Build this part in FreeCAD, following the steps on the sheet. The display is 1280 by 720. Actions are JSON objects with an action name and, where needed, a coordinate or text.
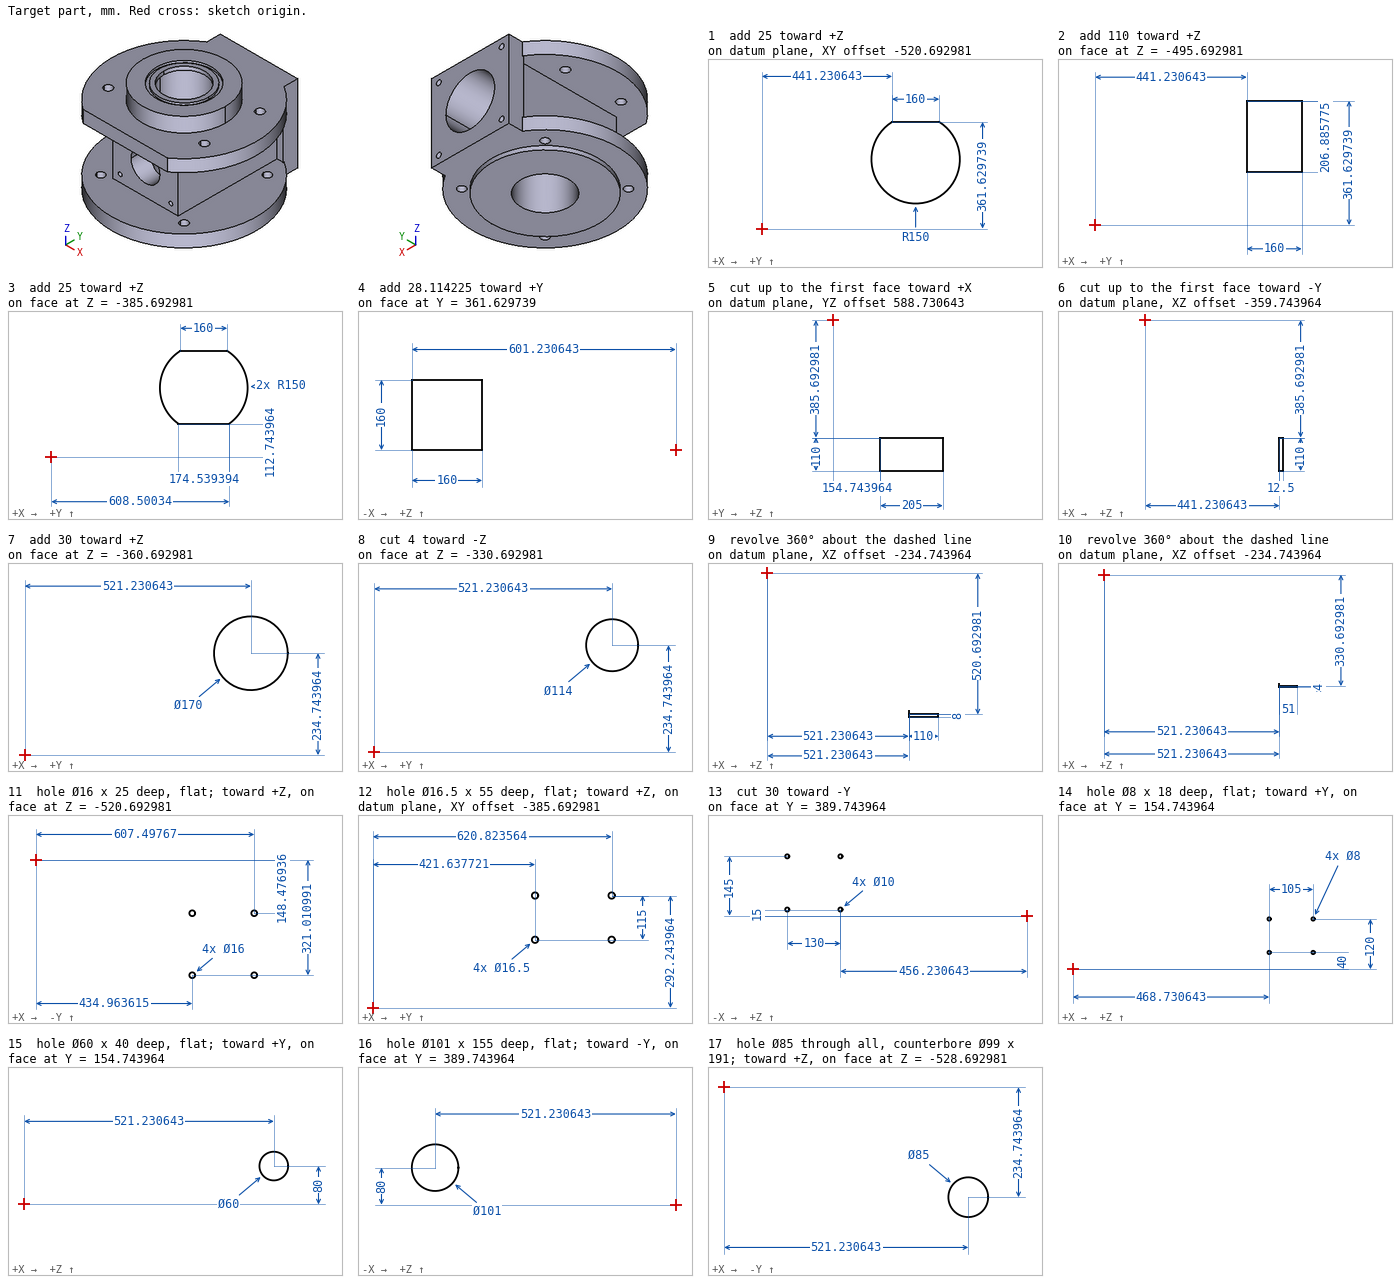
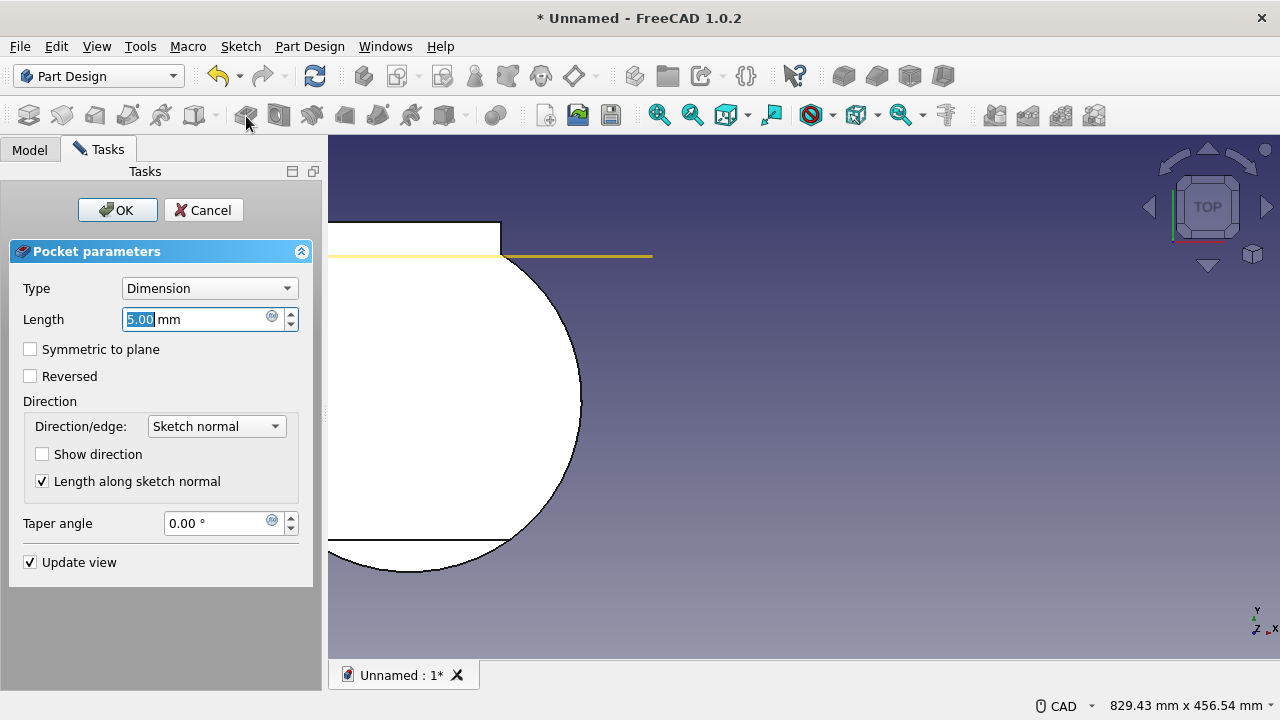
{"action": "left_click", "coordinate": [210, 288]}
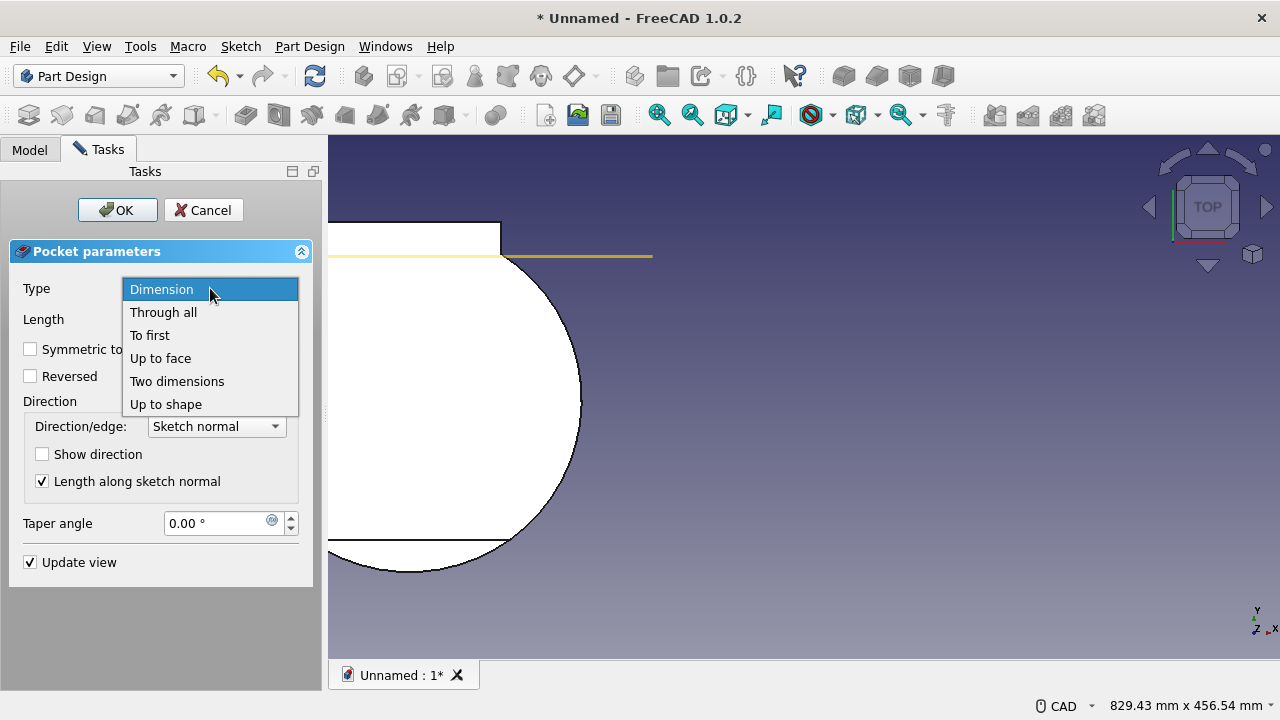
{"action": "left_click", "coordinate": [208, 336]}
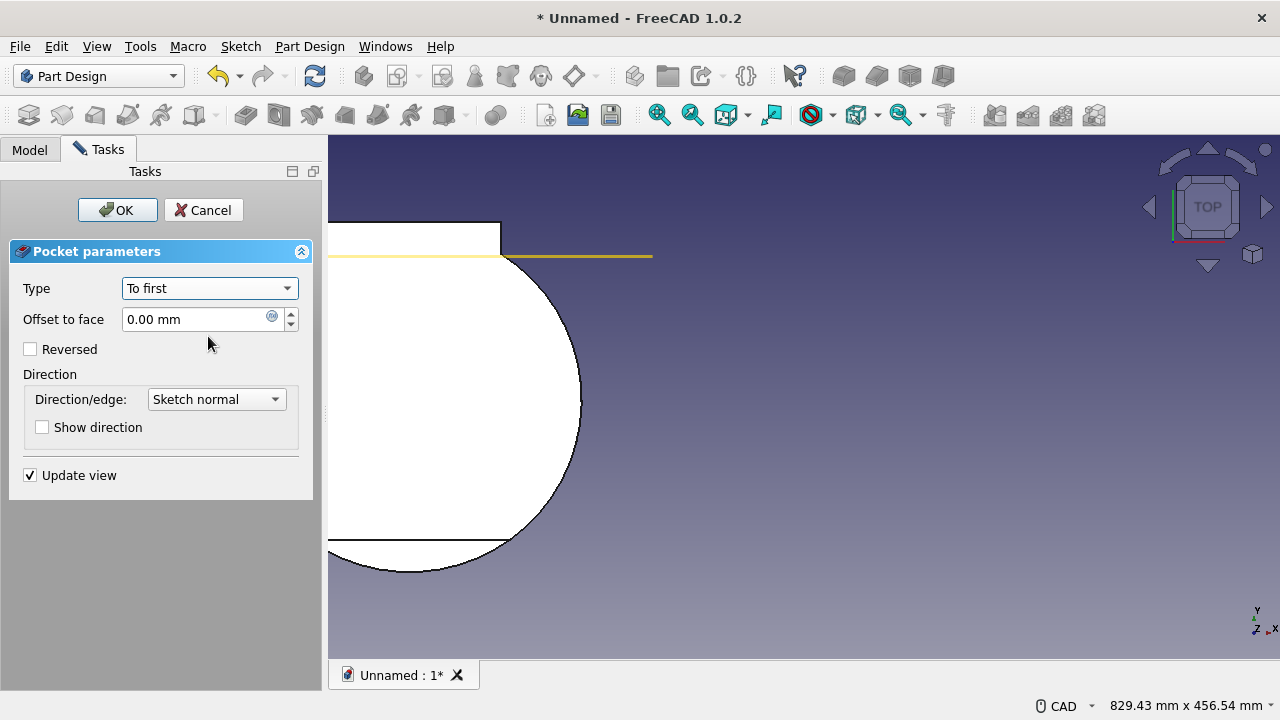
{"action": "left_click", "coordinate": [31, 349]}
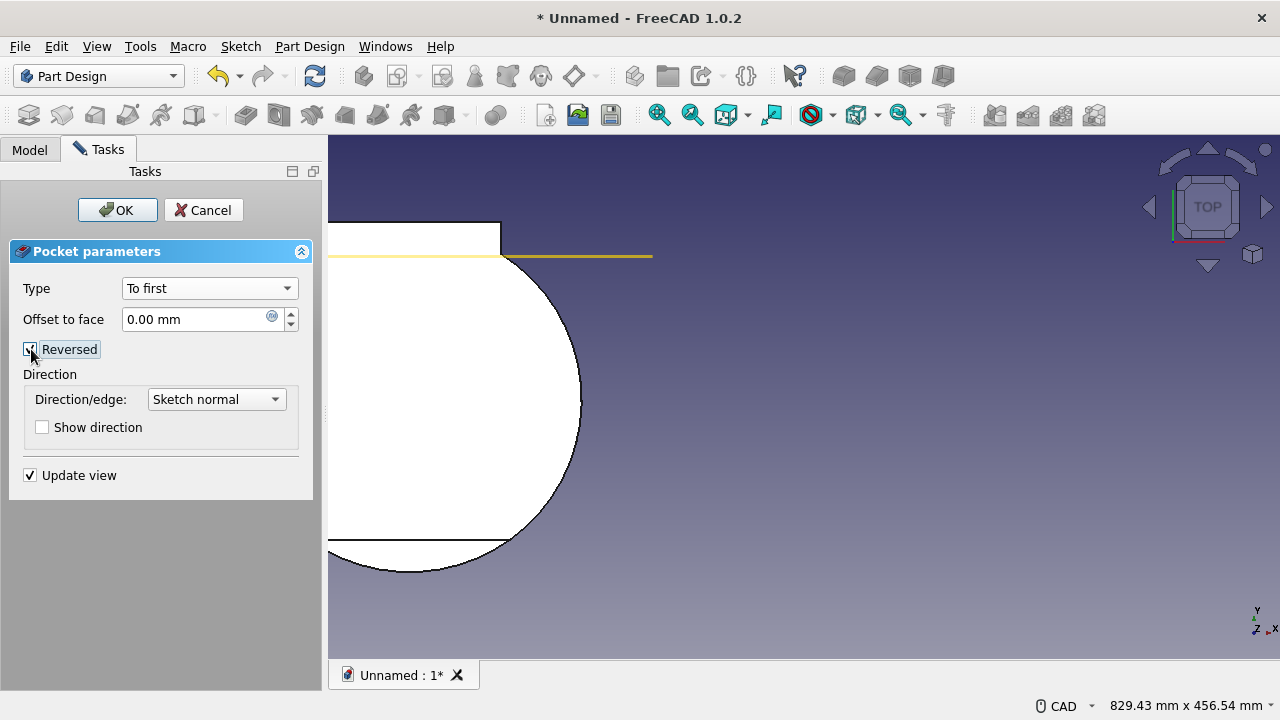
{"action": "left_click", "coordinate": [118, 210]}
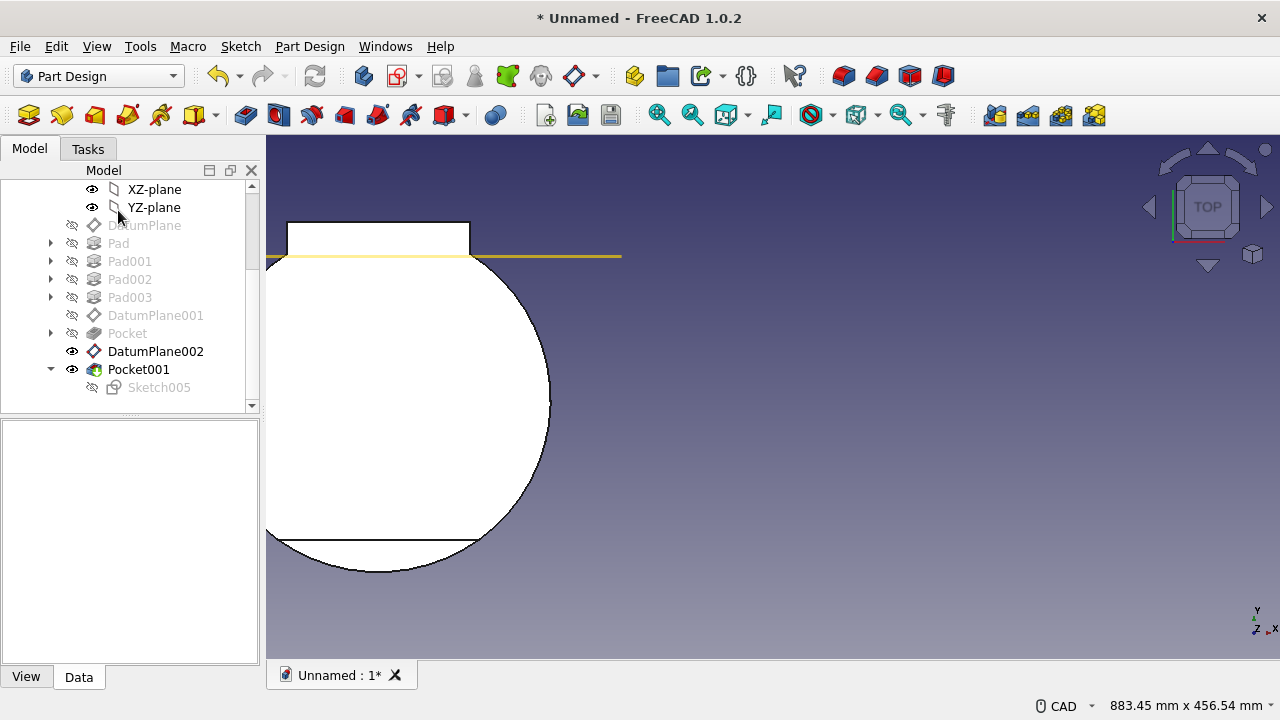
{"action": "left_click", "coordinate": [117, 351]}
{"action": "key", "text": "space"}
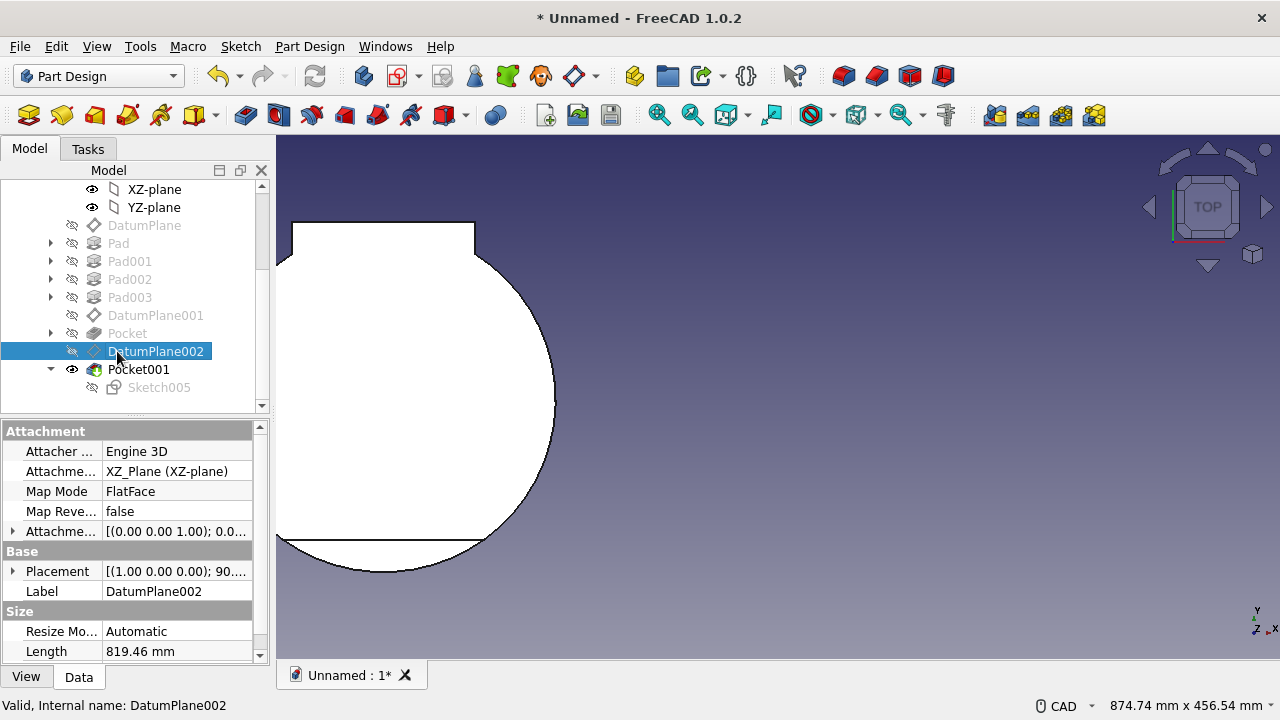
{"action": "left_click", "coordinate": [660, 116]}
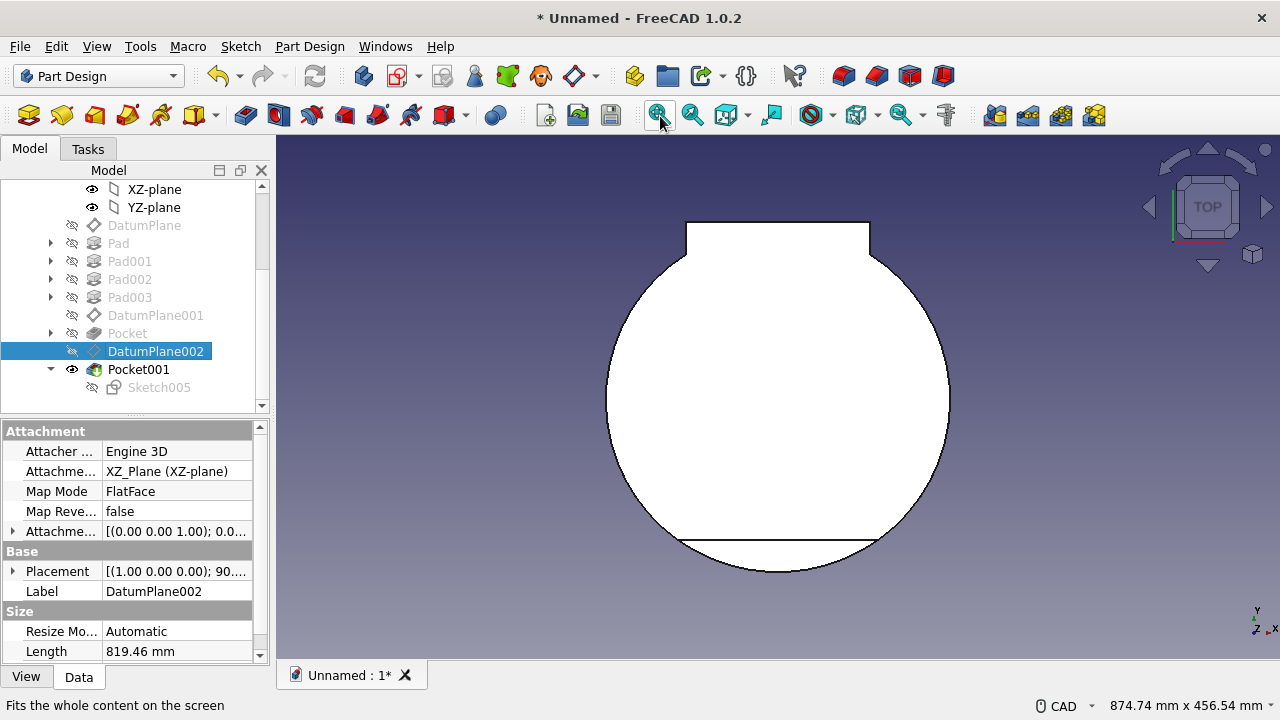
{"action": "left_click", "coordinate": [778, 380]}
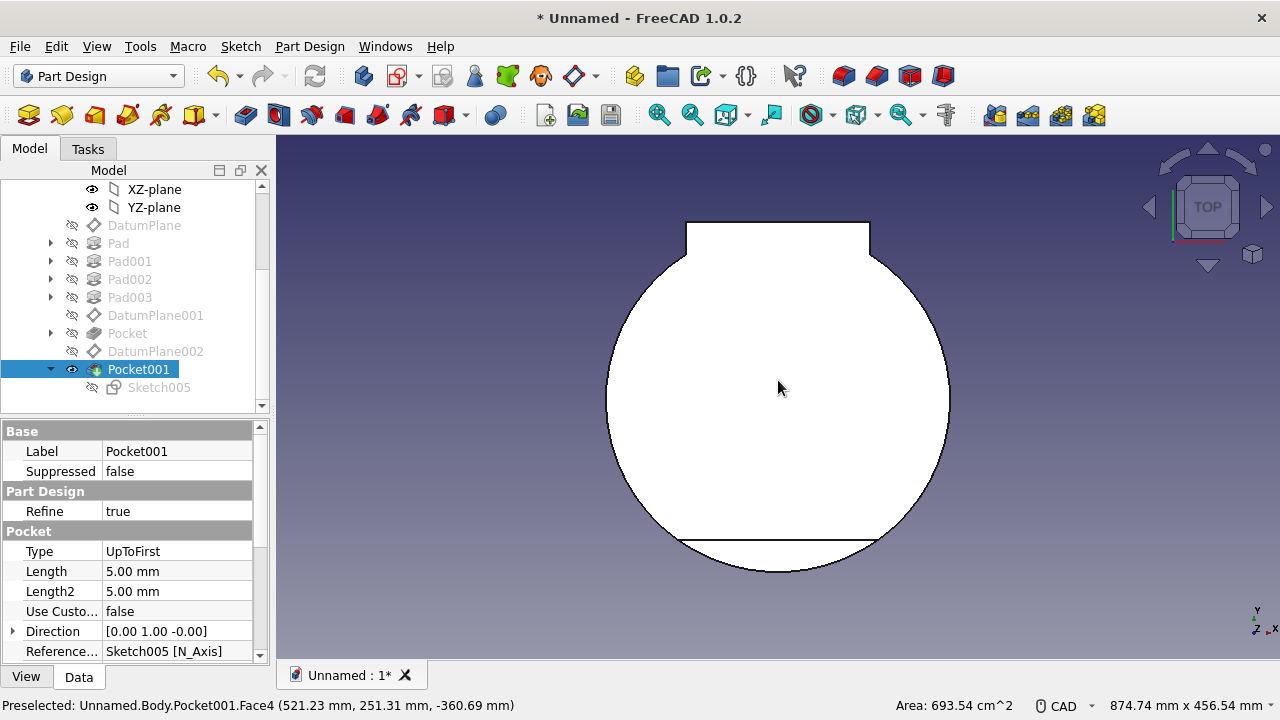
{"action": "left_click", "coordinate": [396, 76]}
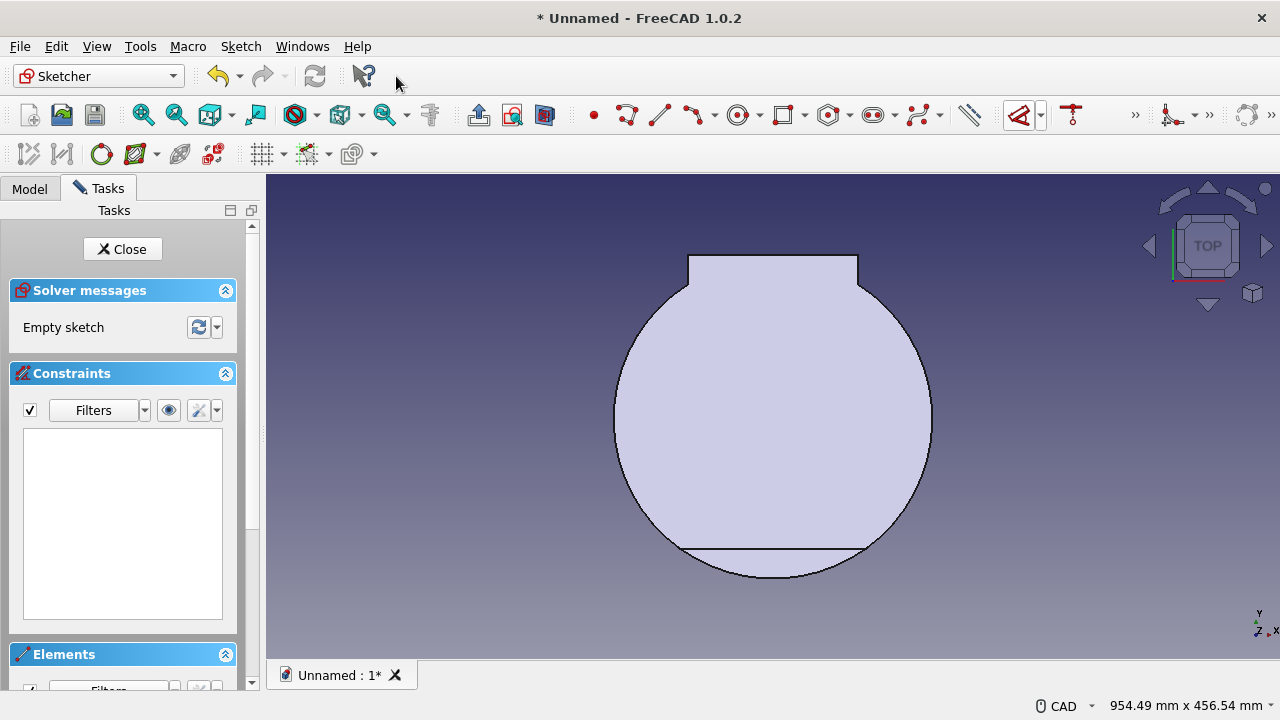
{"action": "scroll", "coordinate": [856, 423], "scroll_direction": "up", "scroll_amount": 3}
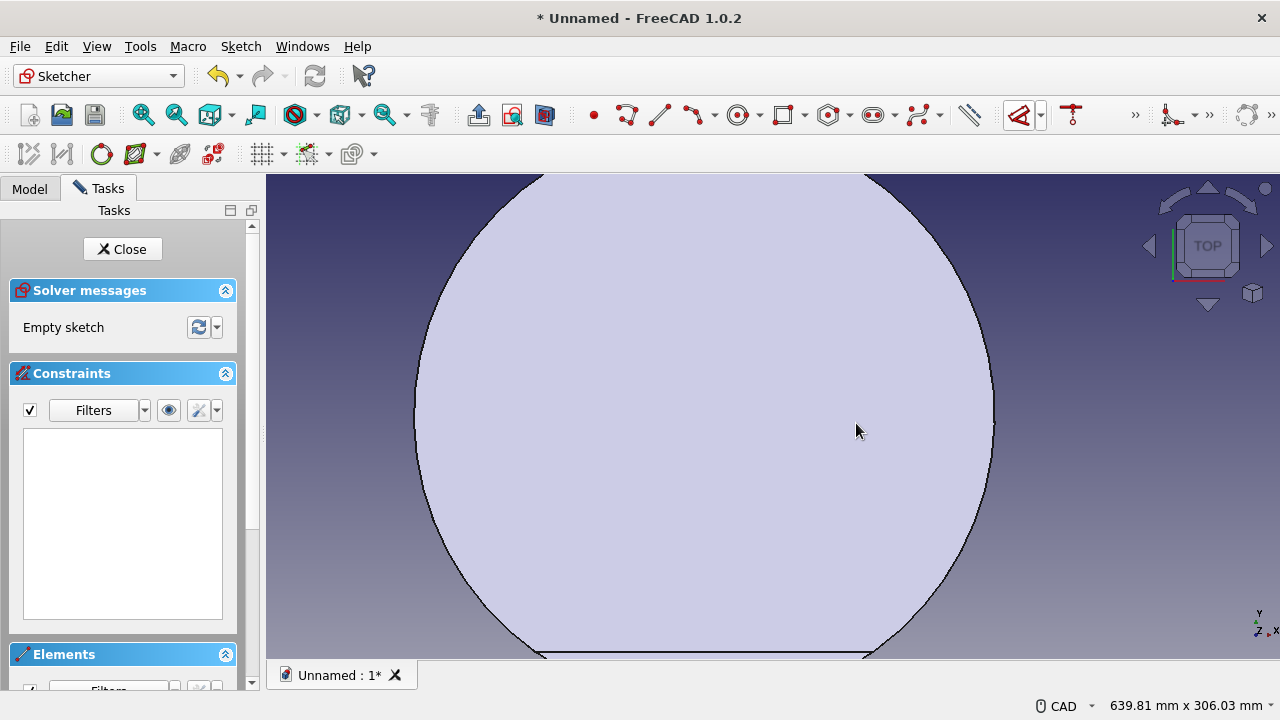
{"action": "left_click", "coordinate": [738, 116]}